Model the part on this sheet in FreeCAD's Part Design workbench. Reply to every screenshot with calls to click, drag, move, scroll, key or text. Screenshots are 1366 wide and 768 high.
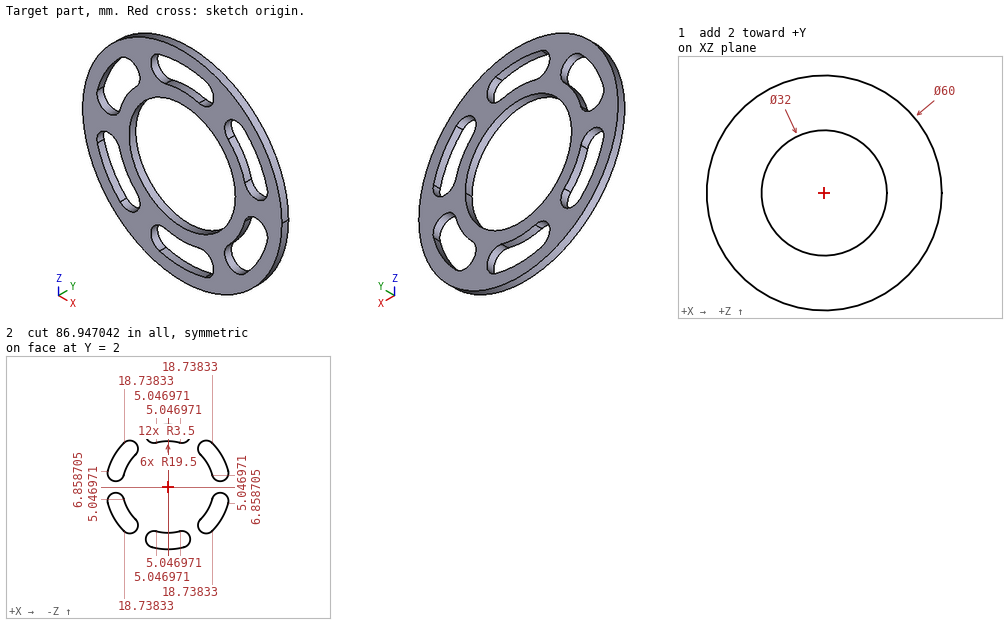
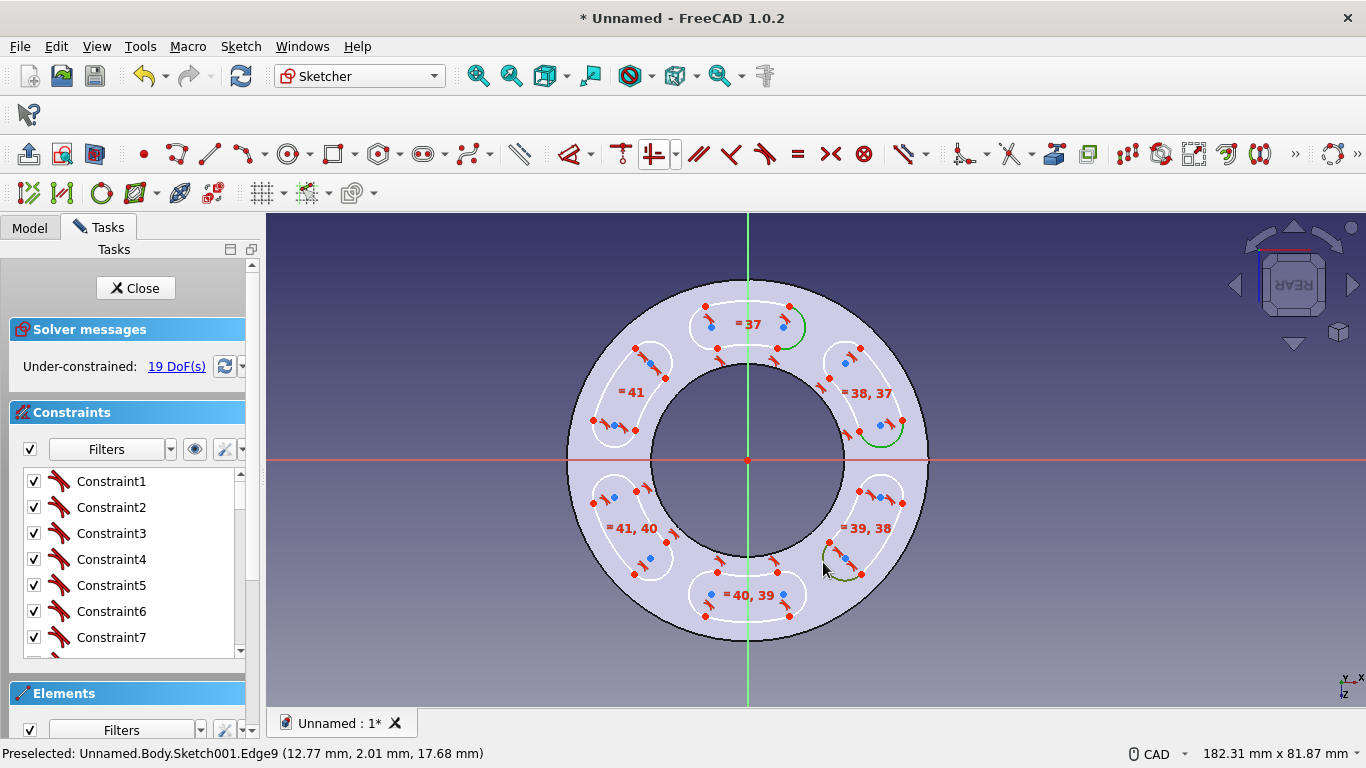
click(697, 577)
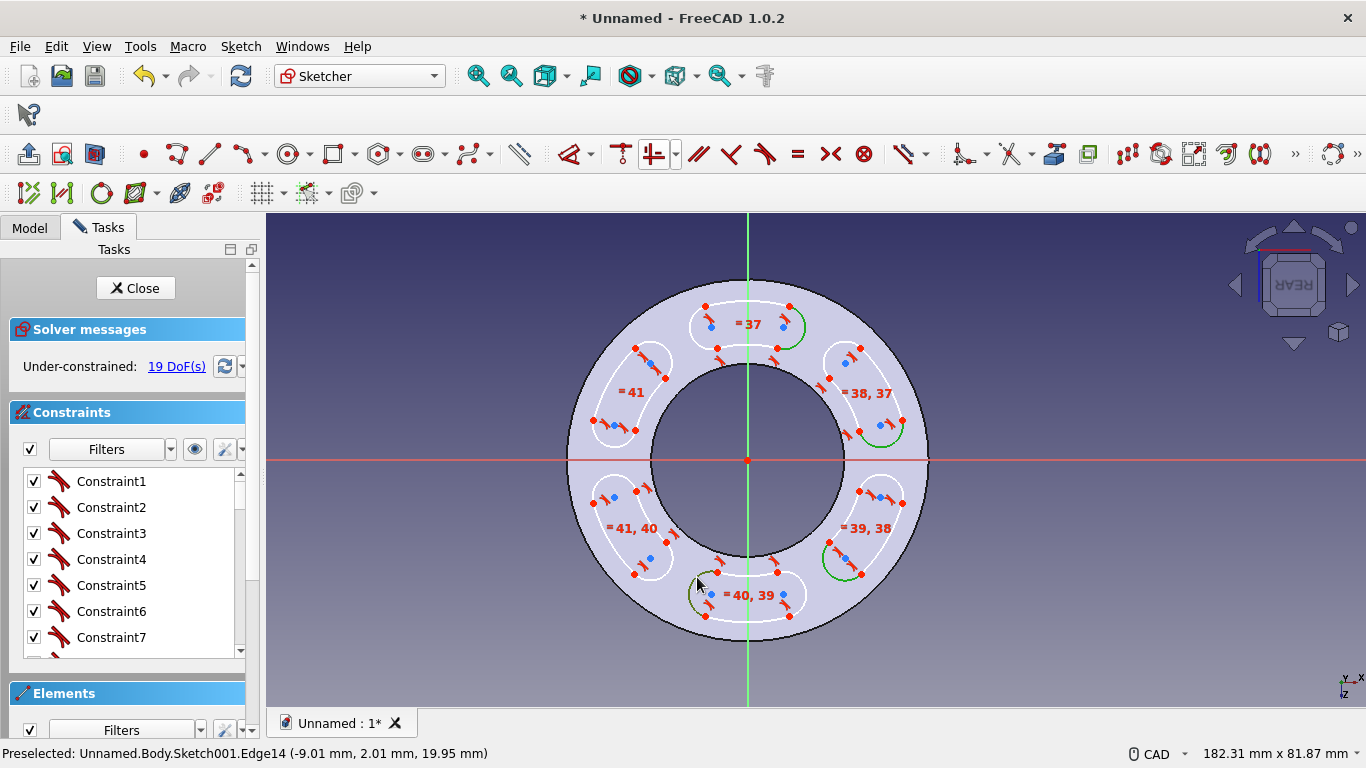
click(623, 476)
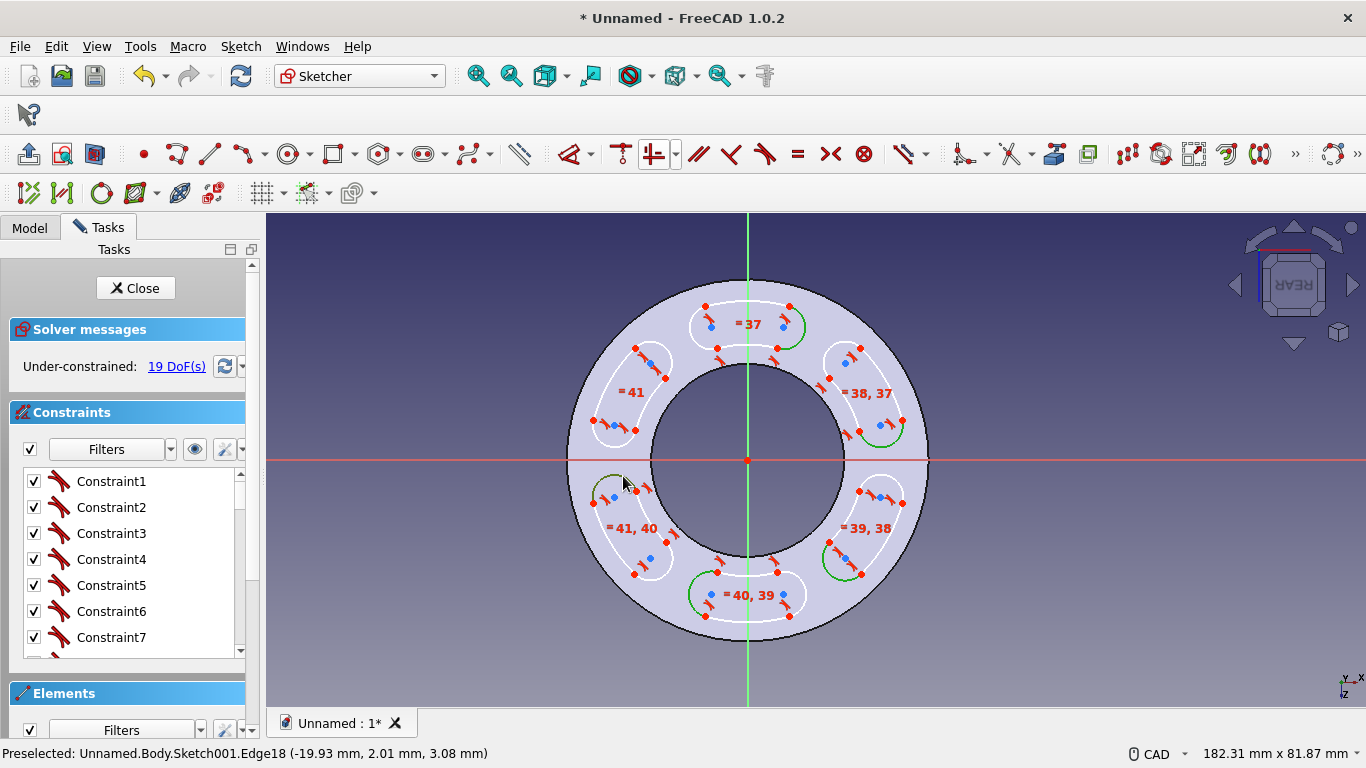
click(672, 360)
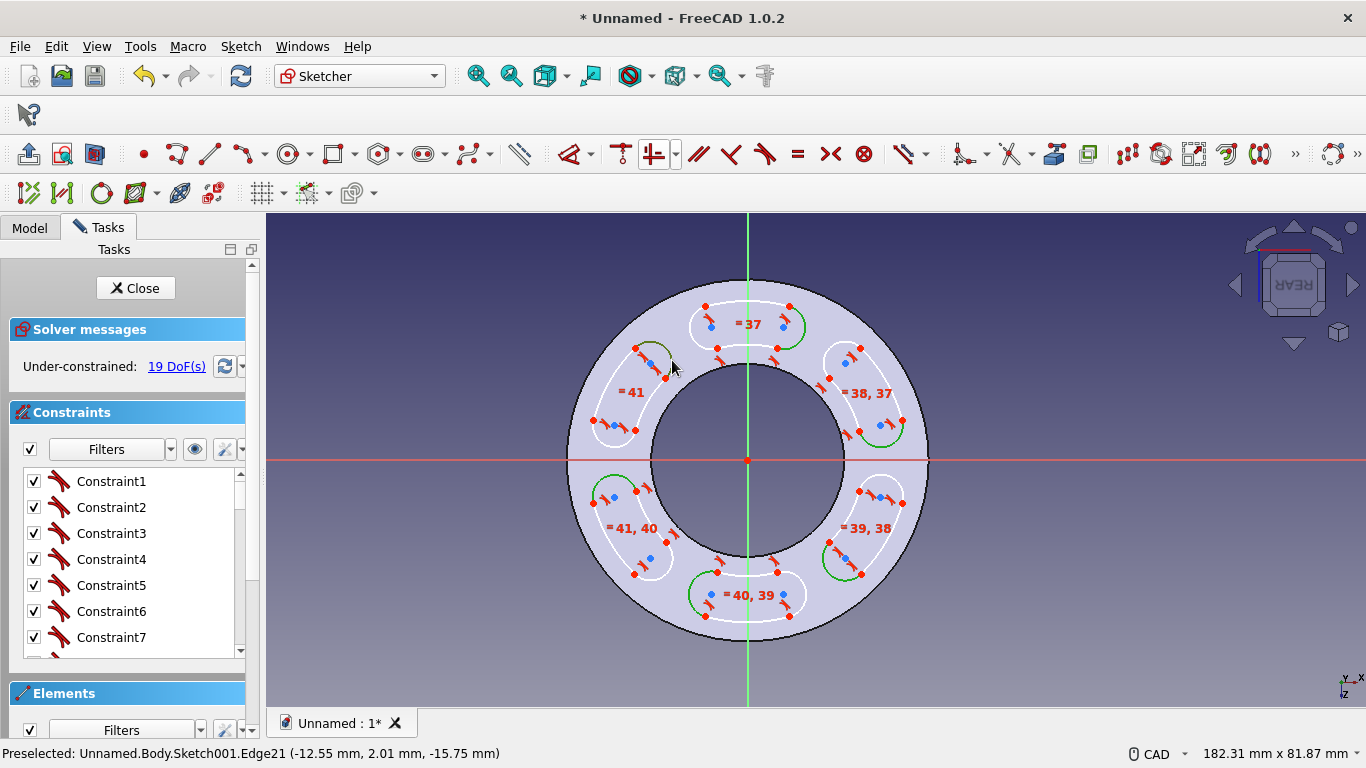
click(798, 154)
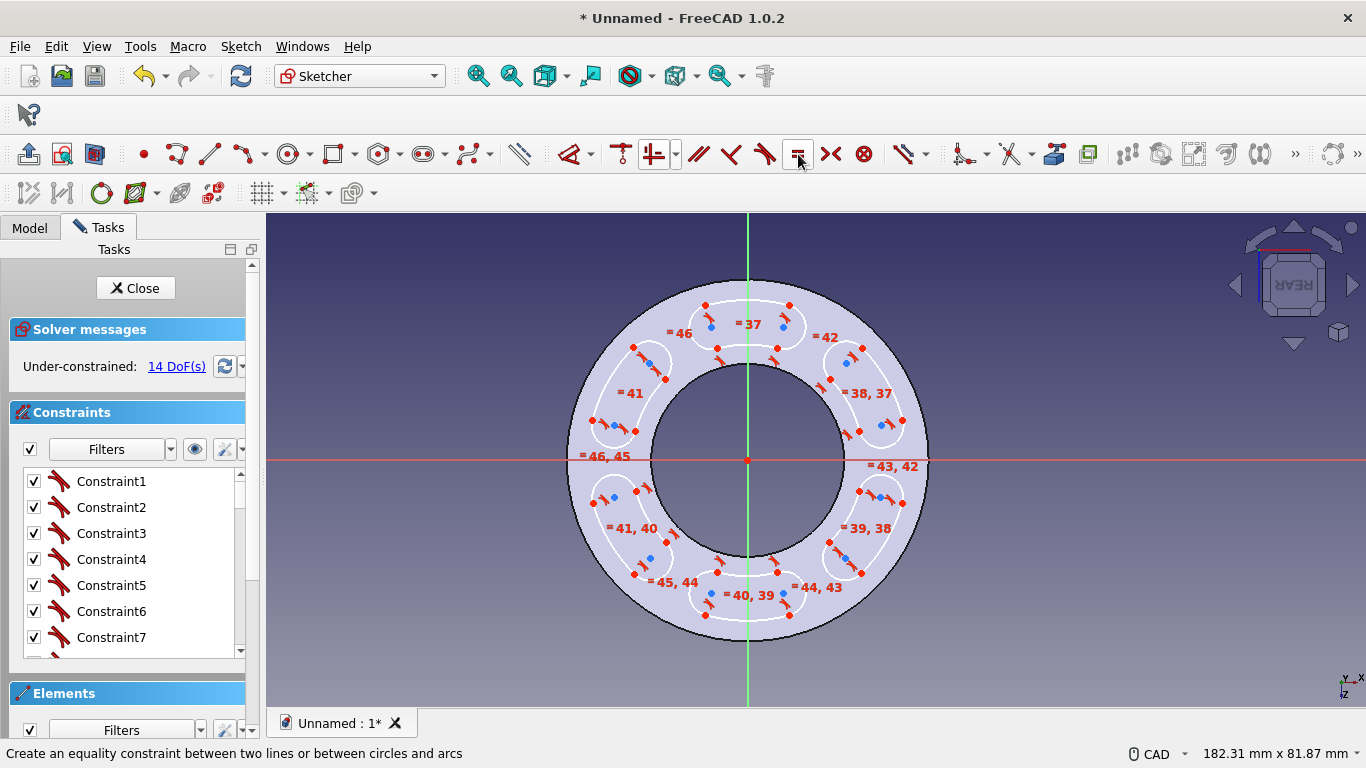
key(d)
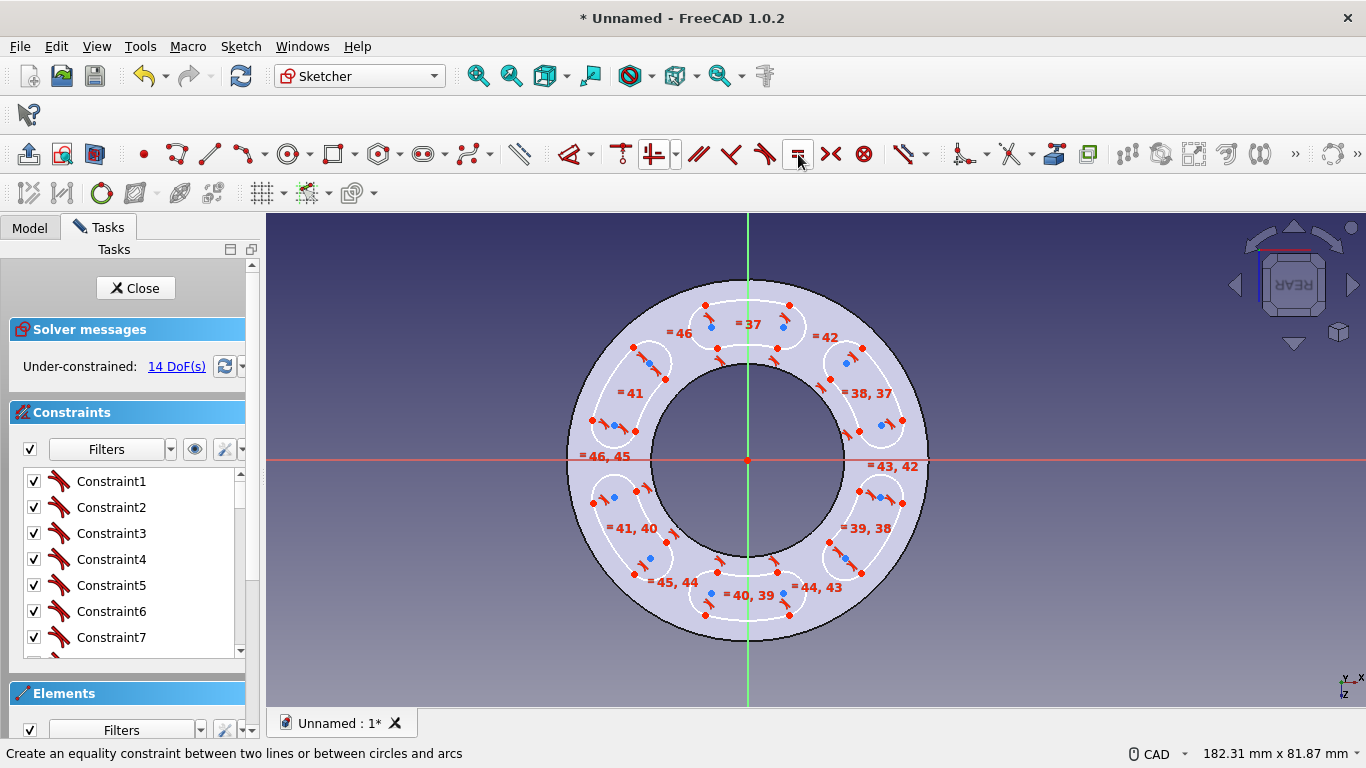
click(760, 345)
click(845, 320)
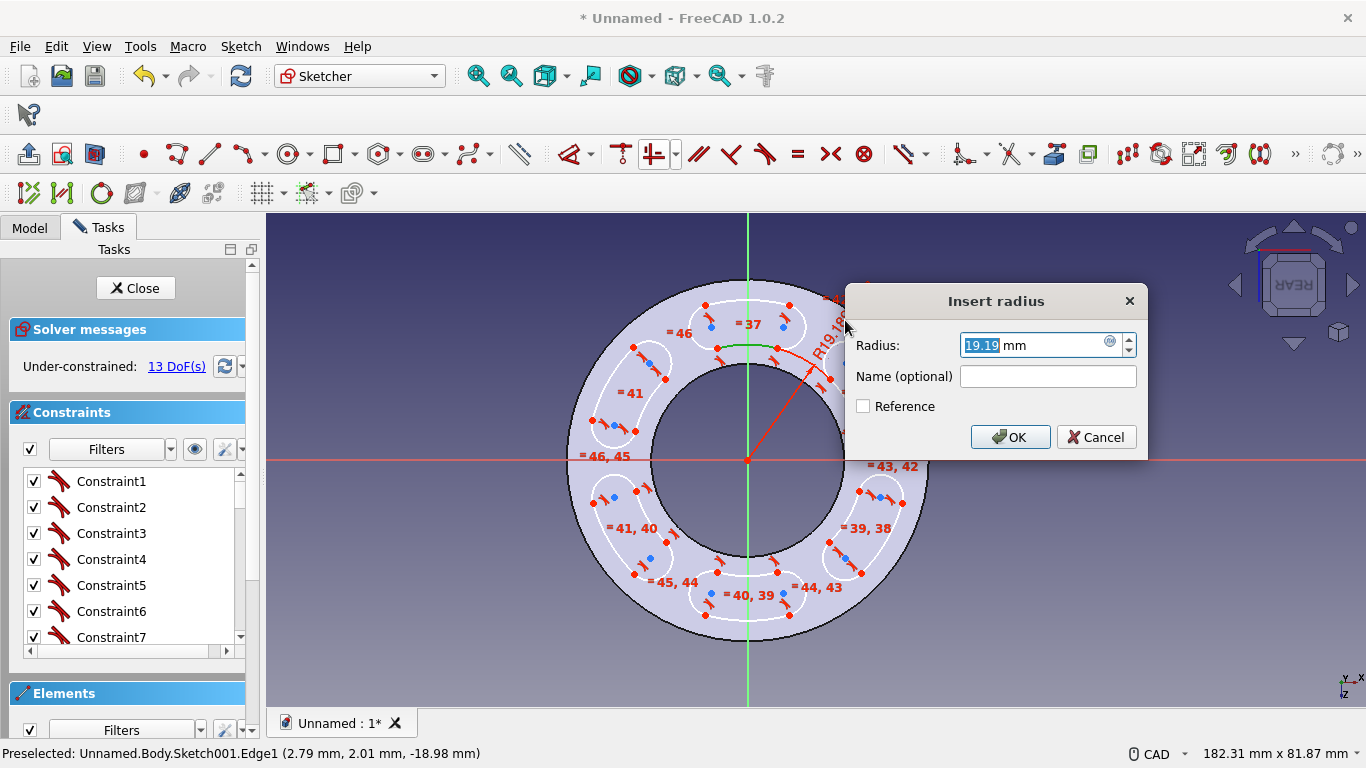
text(19.5)
key(Return)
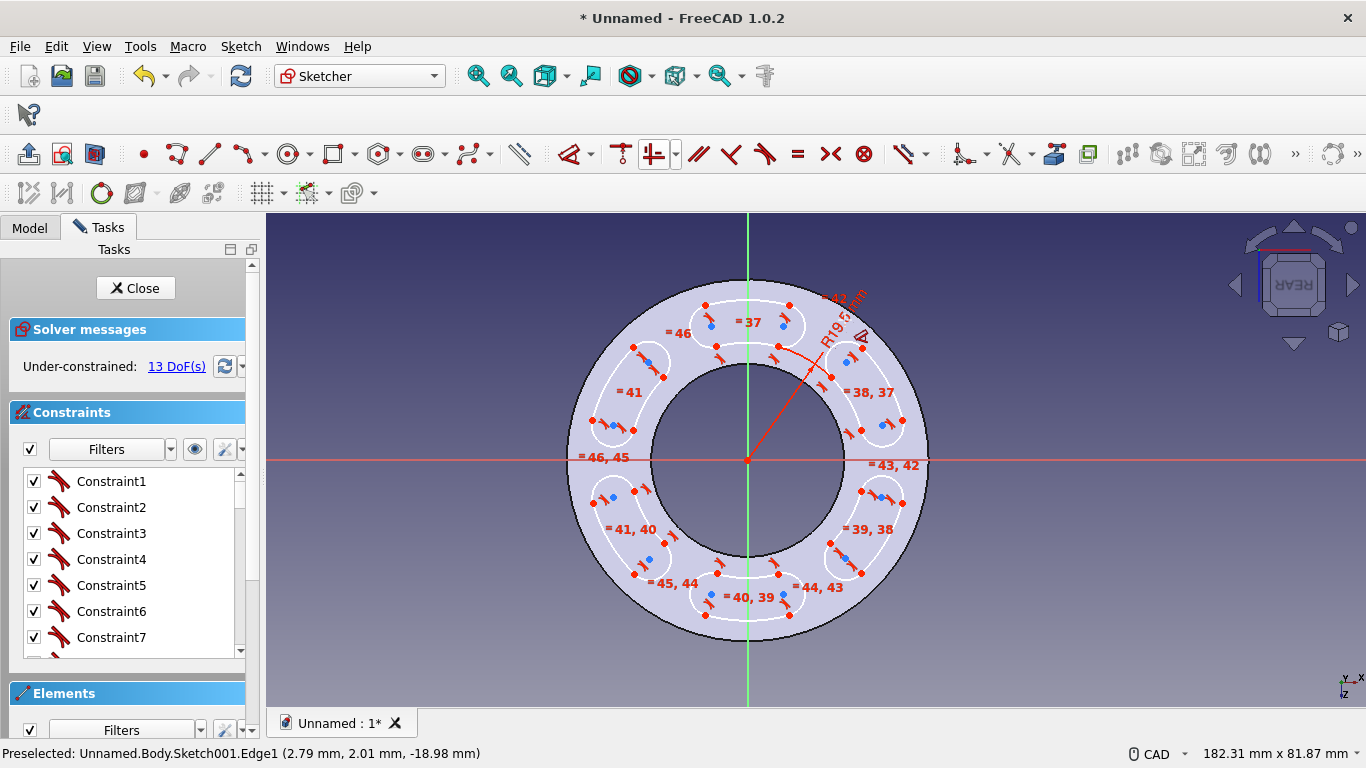
scroll(797, 343, up, 4)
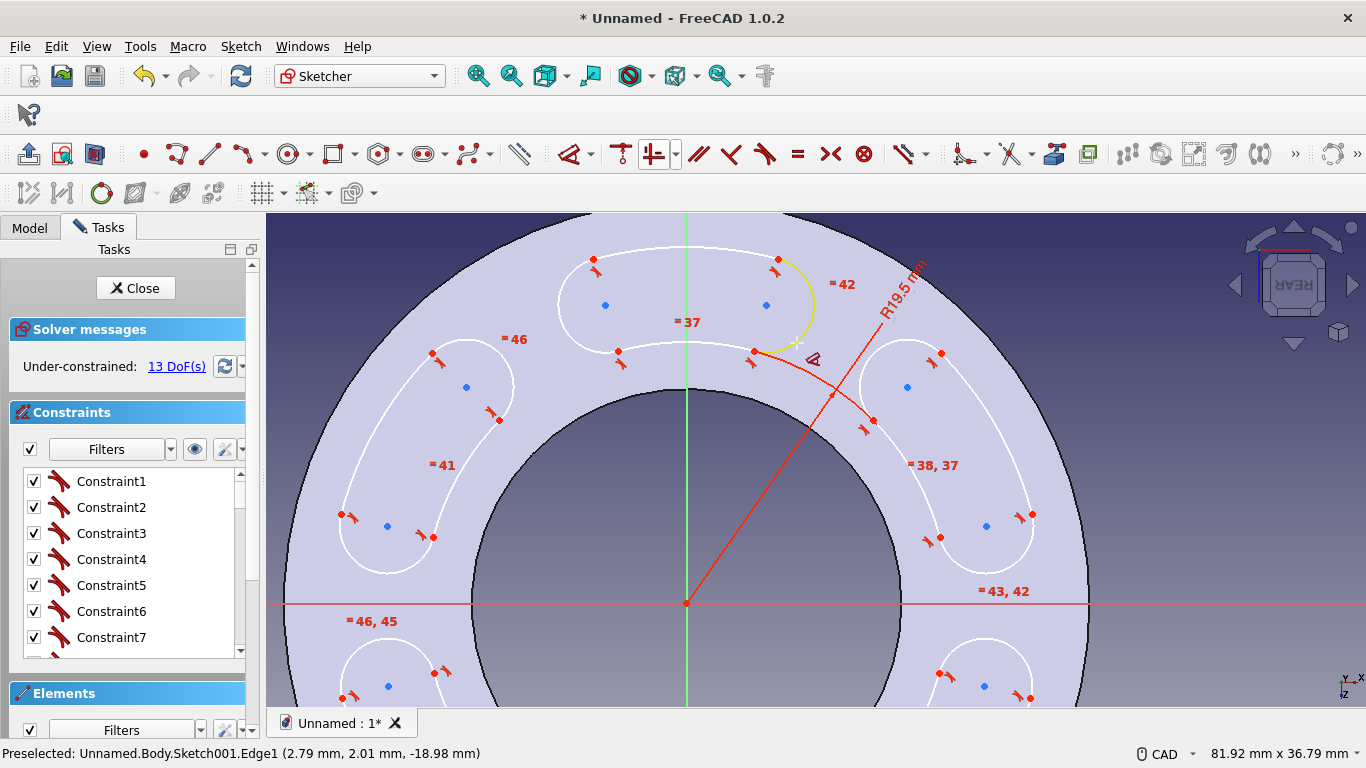
click(797, 342)
click(817, 367)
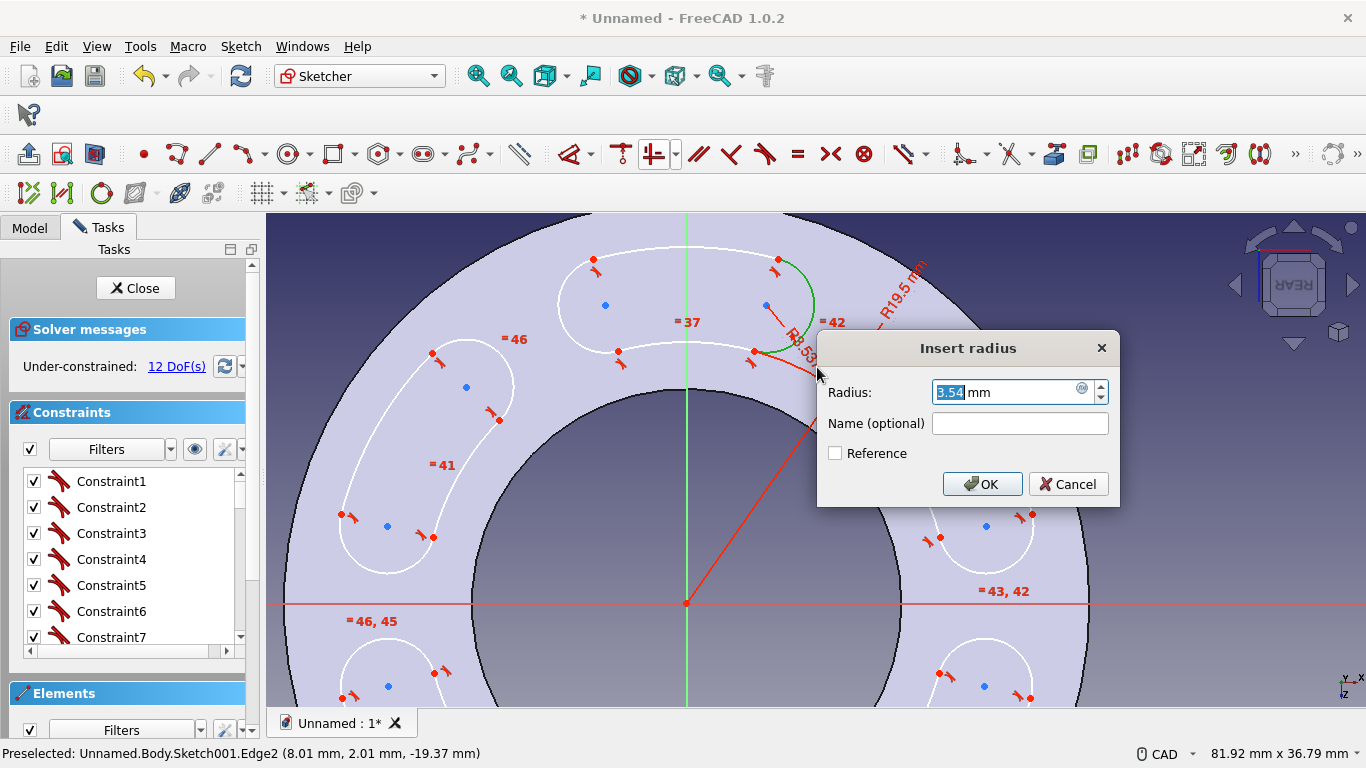
text(3.5)
key(Return)